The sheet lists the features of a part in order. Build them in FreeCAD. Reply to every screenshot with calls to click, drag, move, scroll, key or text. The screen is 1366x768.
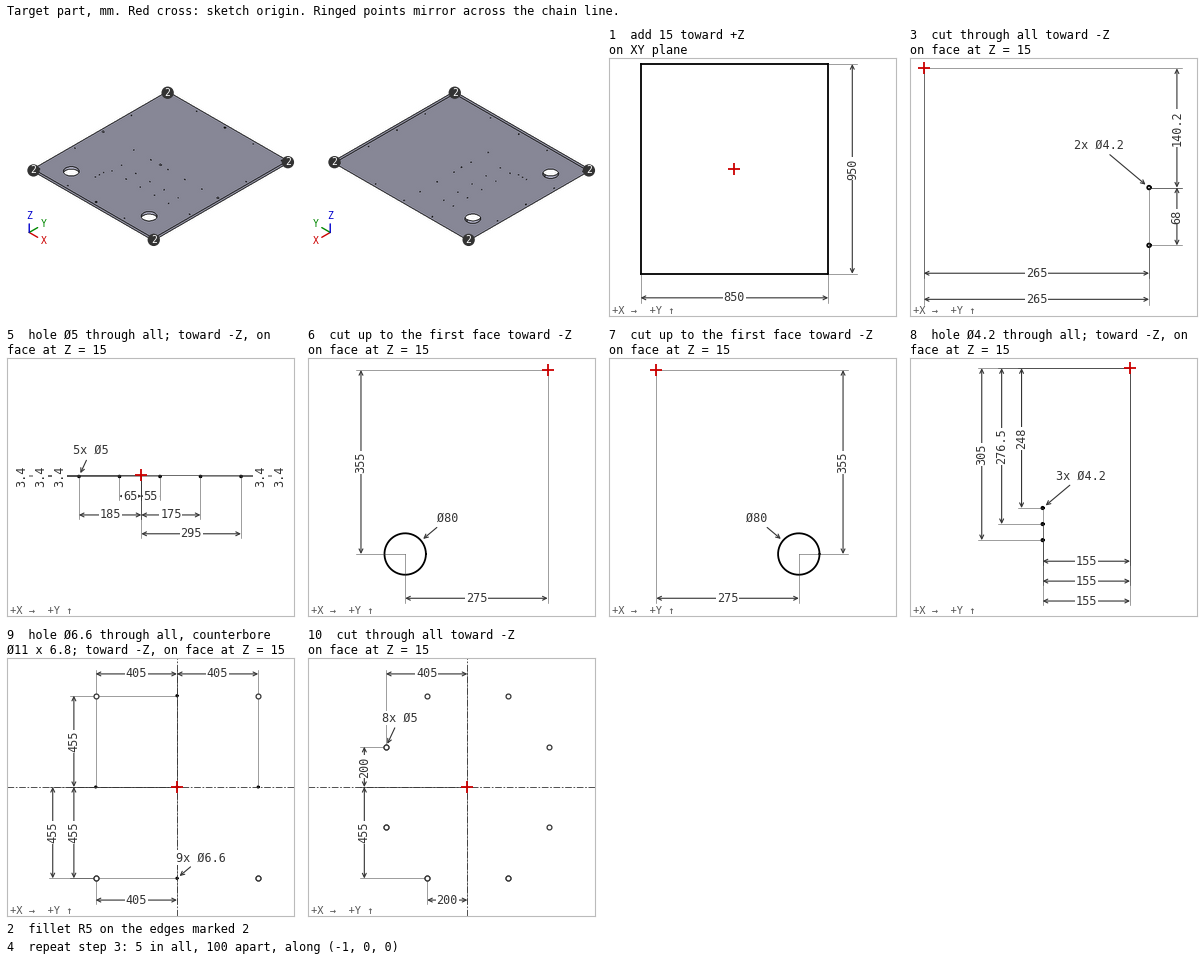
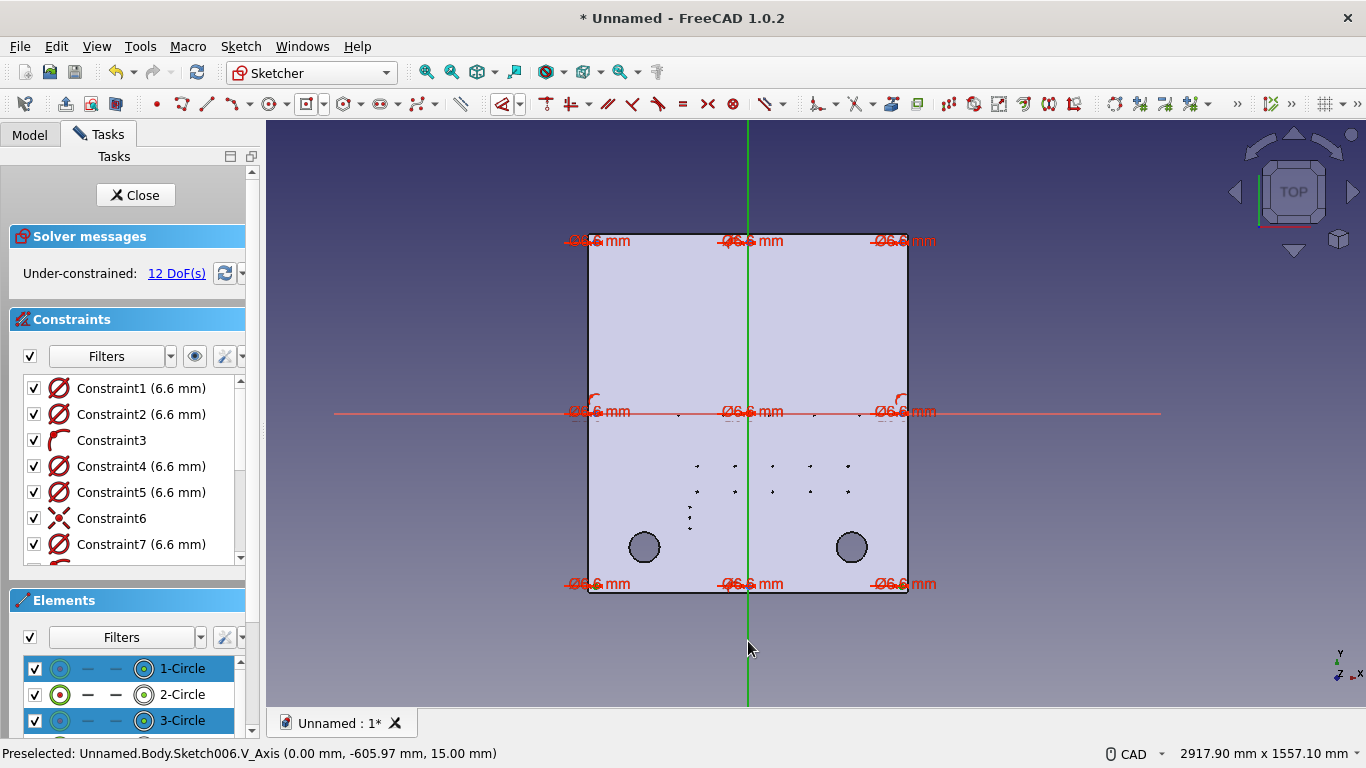
click(708, 104)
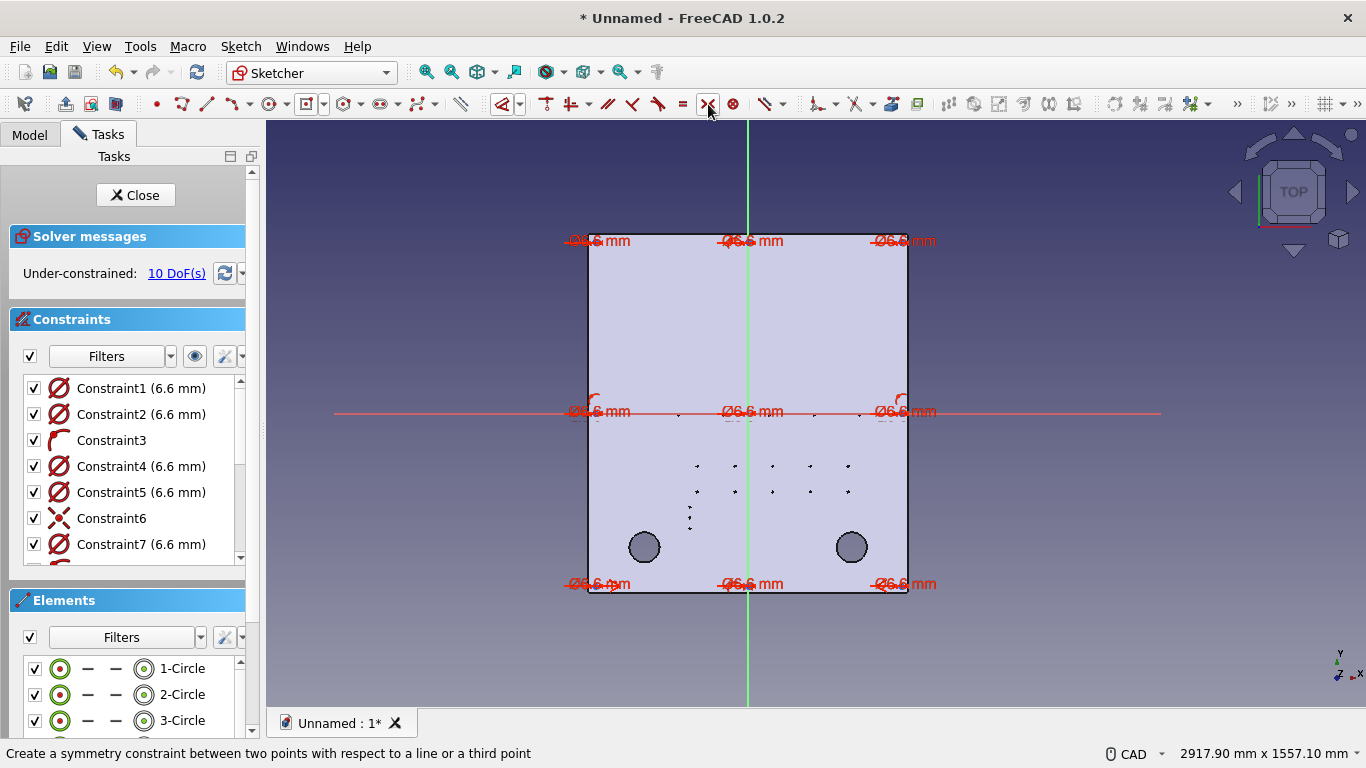
click(595, 586)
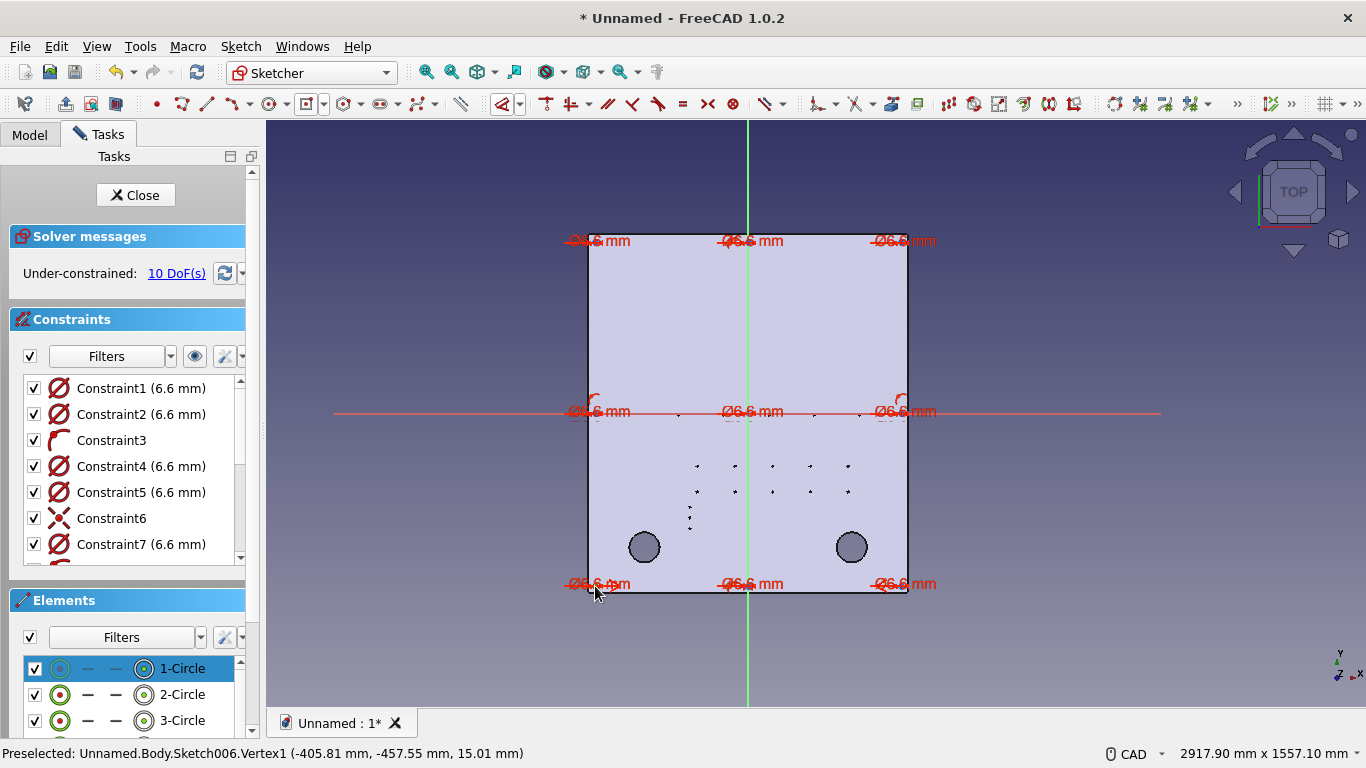
click(595, 243)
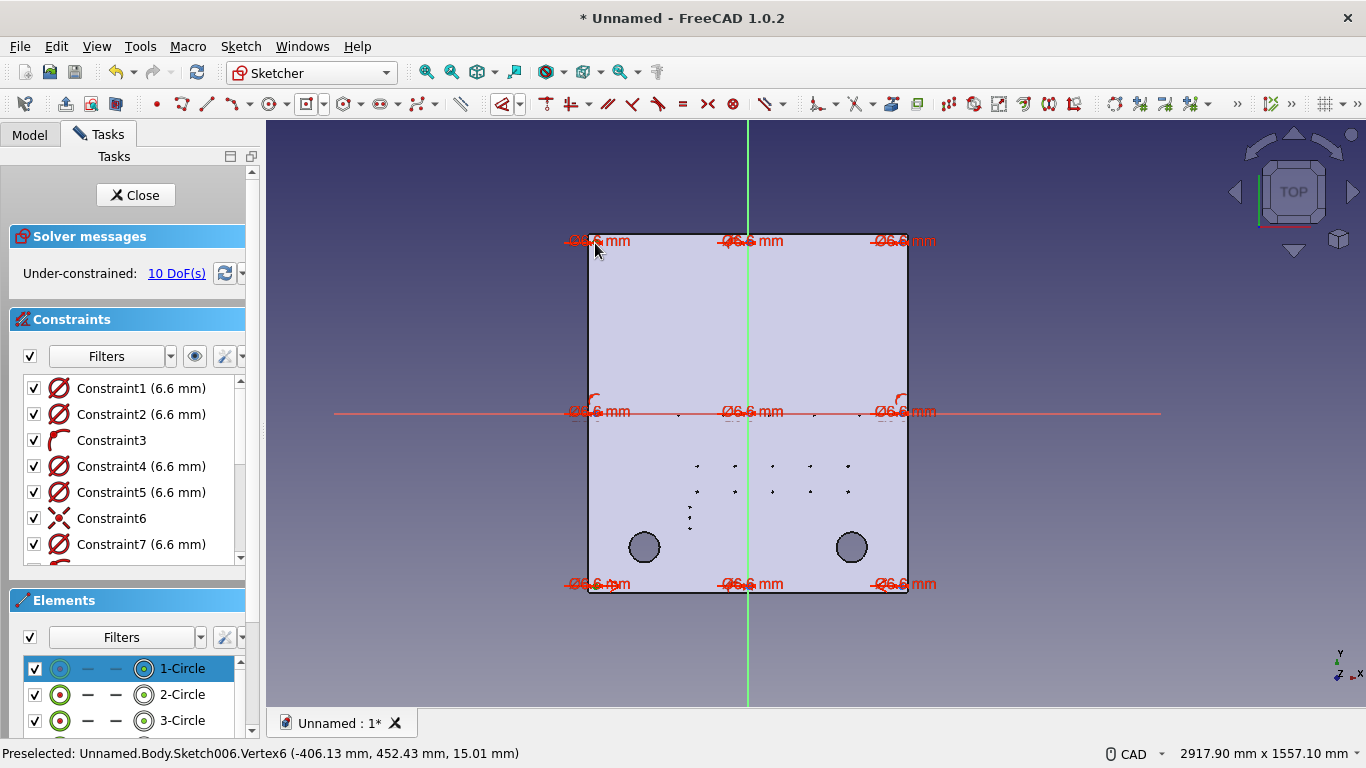
click(359, 414)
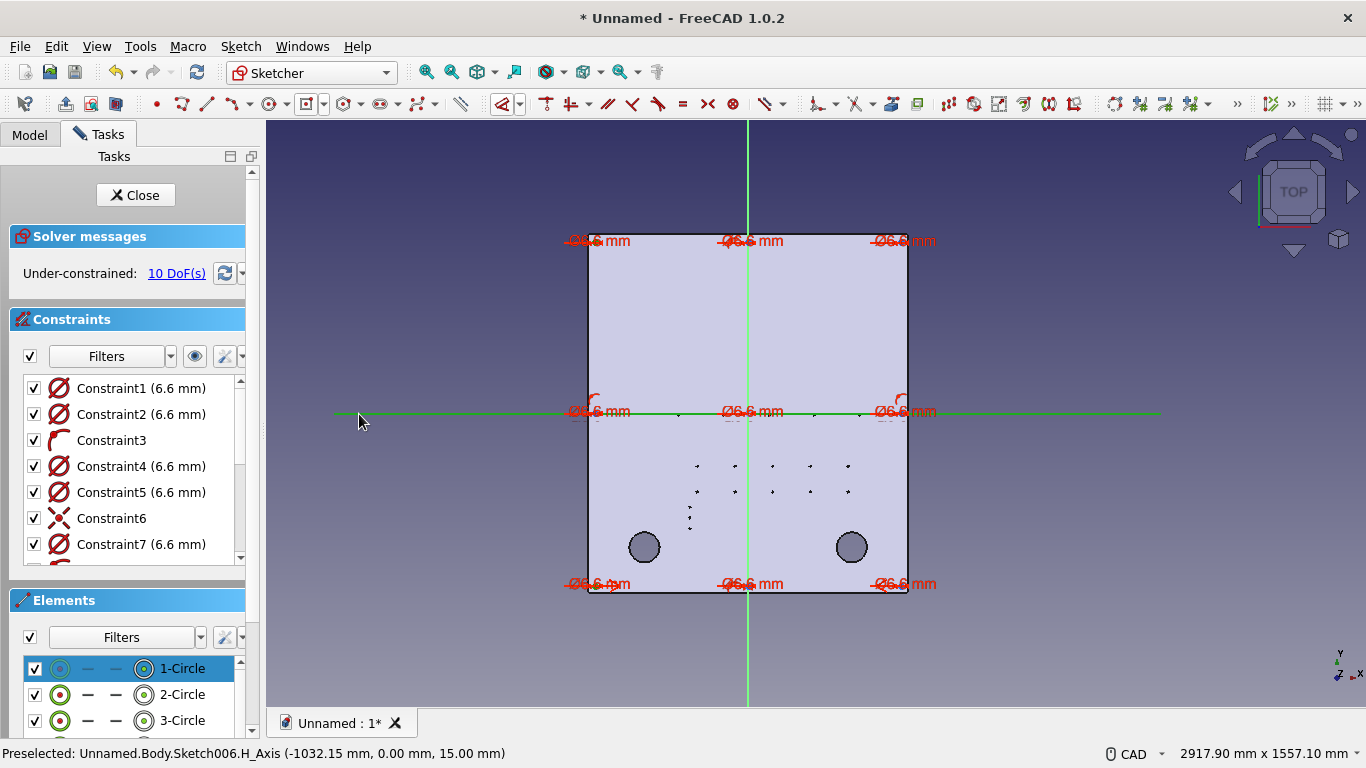
click(708, 104)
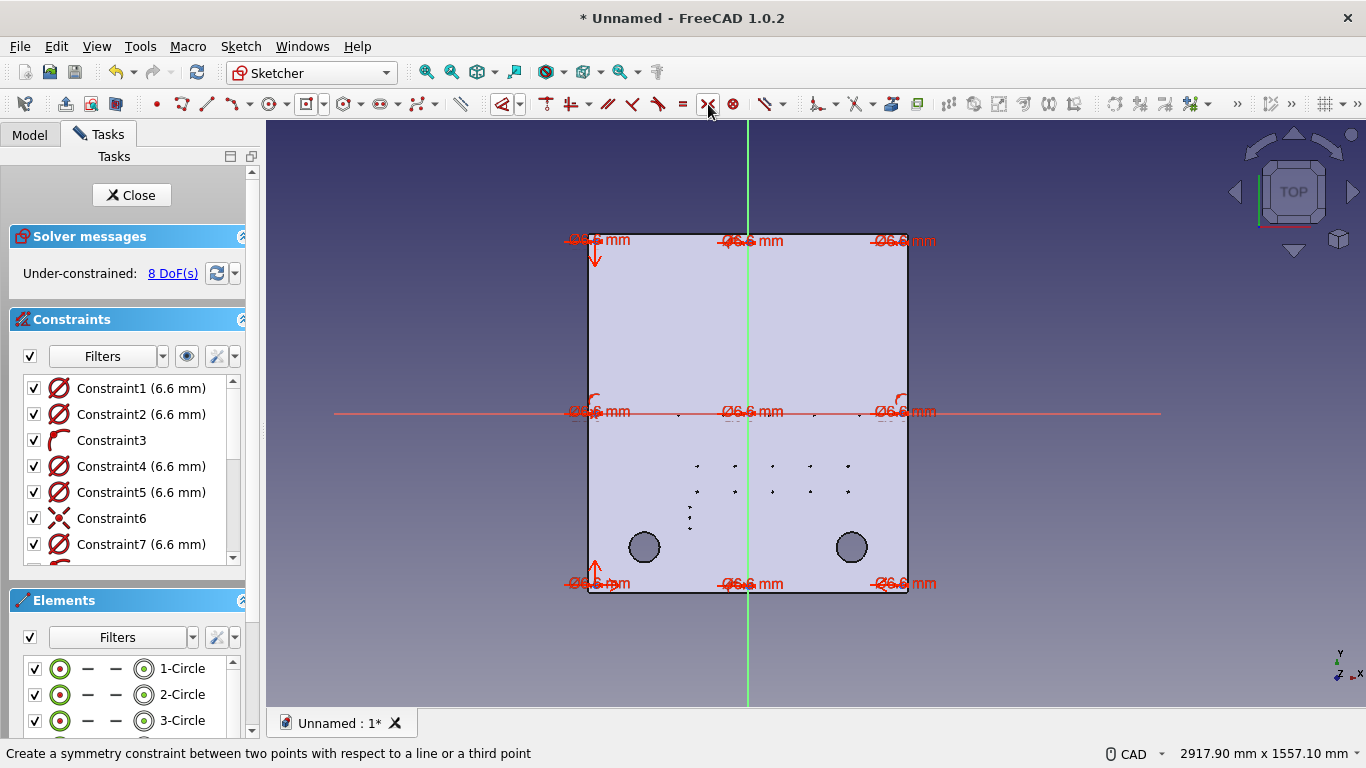
click(901, 585)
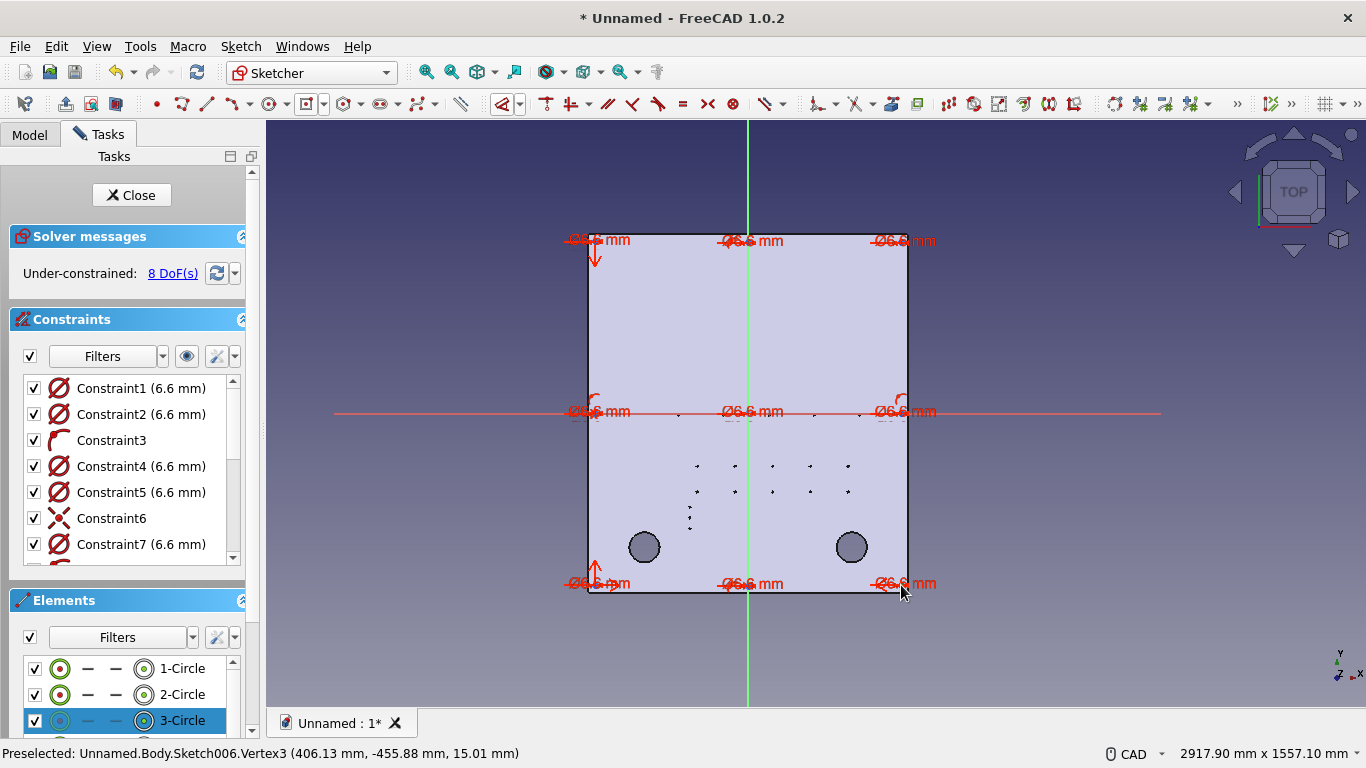
click(901, 243)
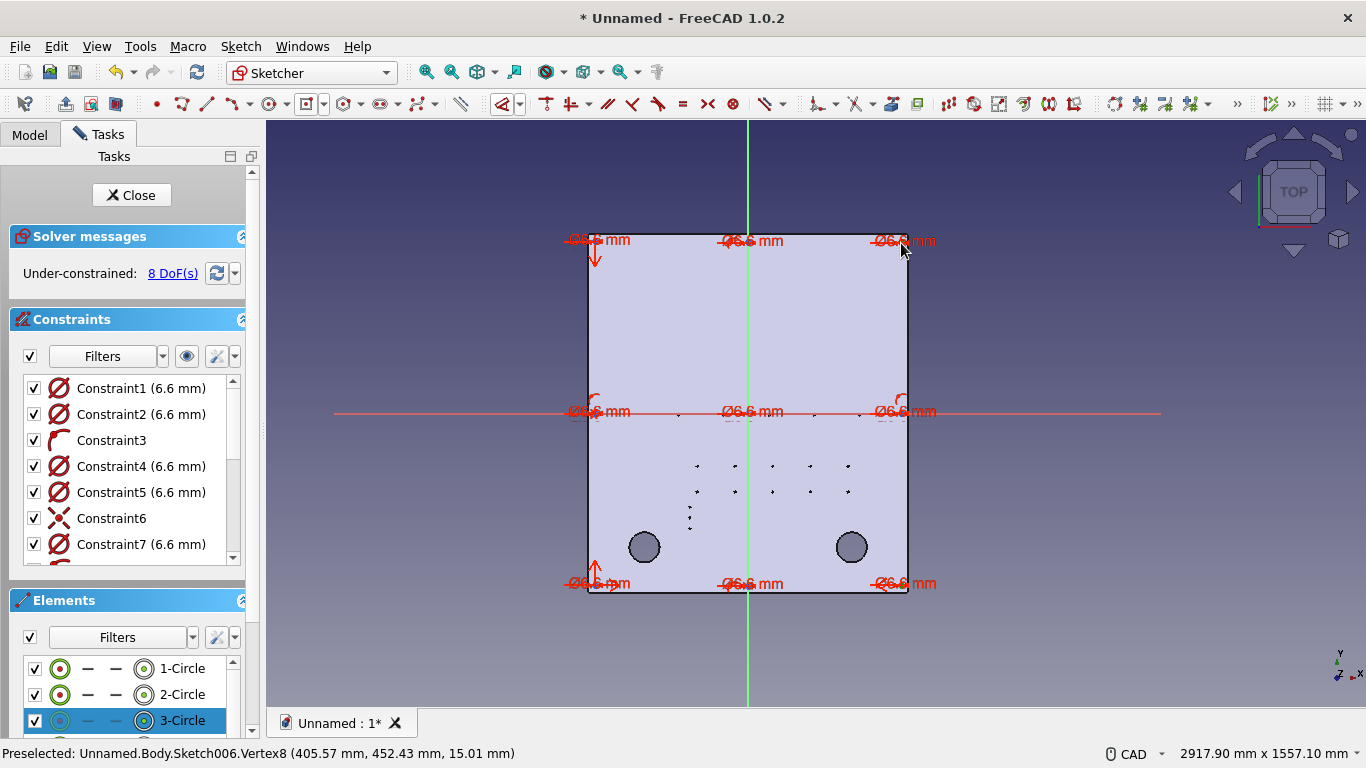
click(359, 414)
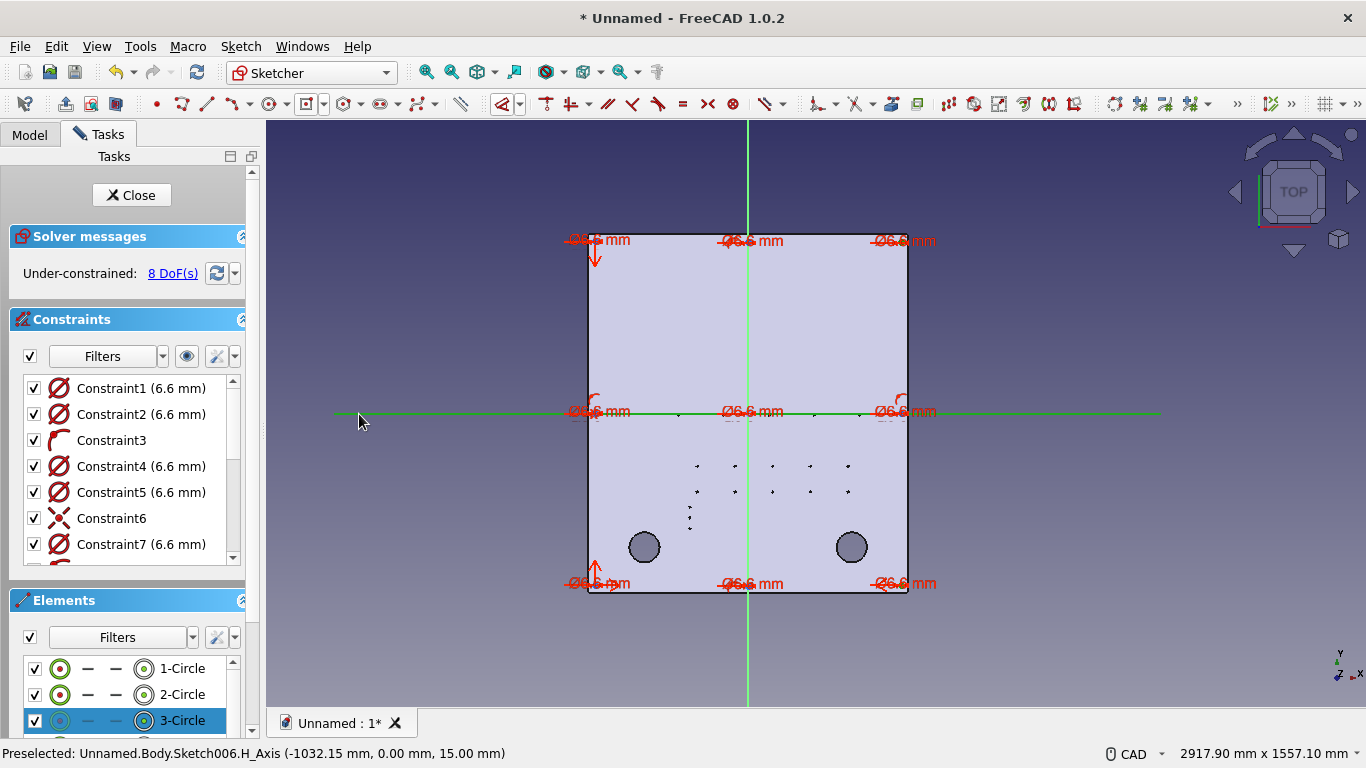
click(708, 104)